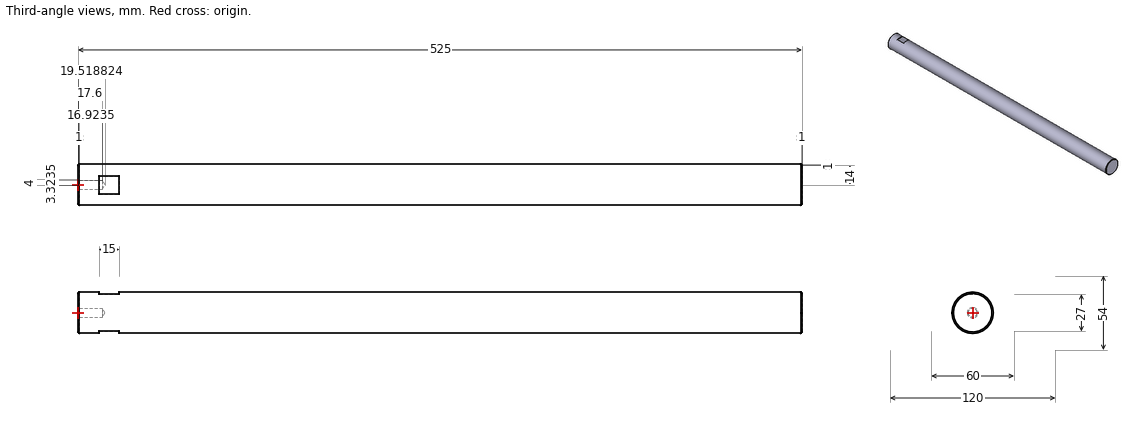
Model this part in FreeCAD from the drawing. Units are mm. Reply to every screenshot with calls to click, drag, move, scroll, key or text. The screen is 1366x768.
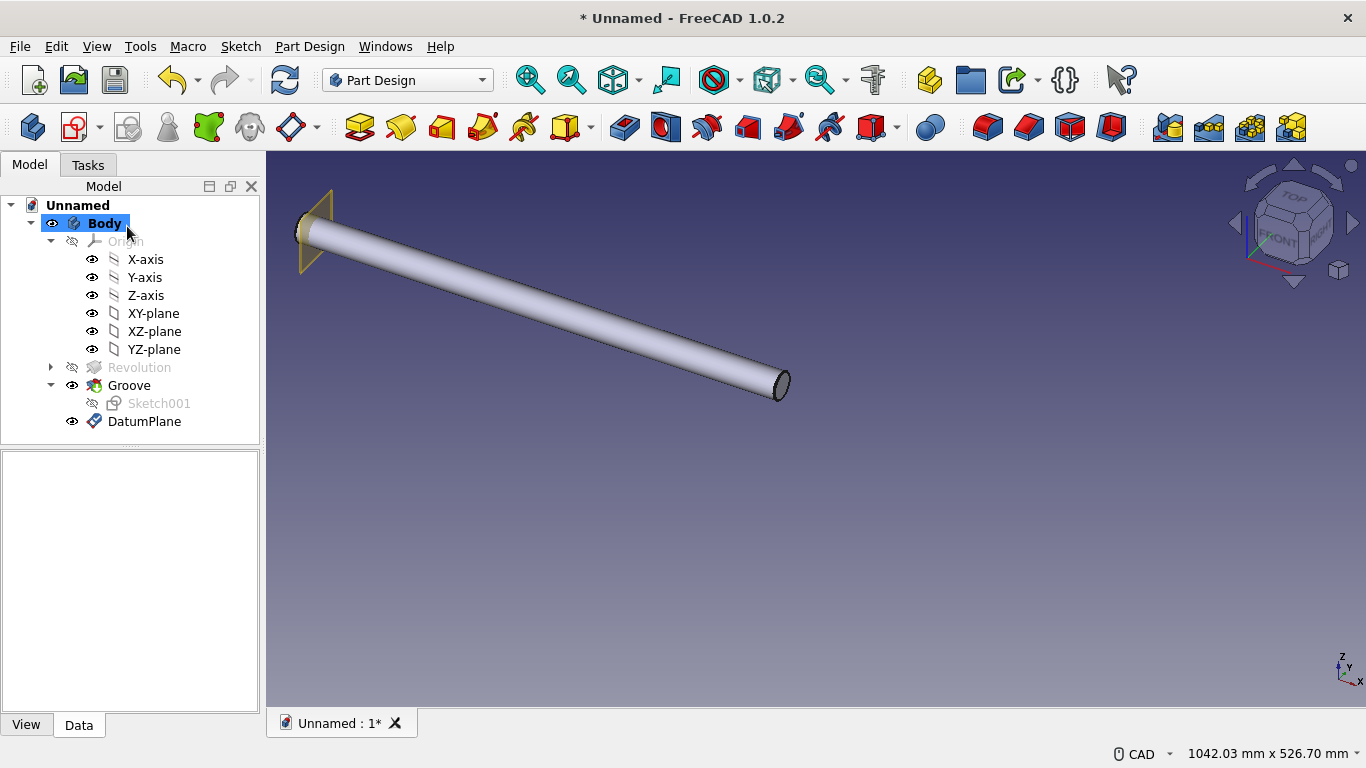
click(117, 421)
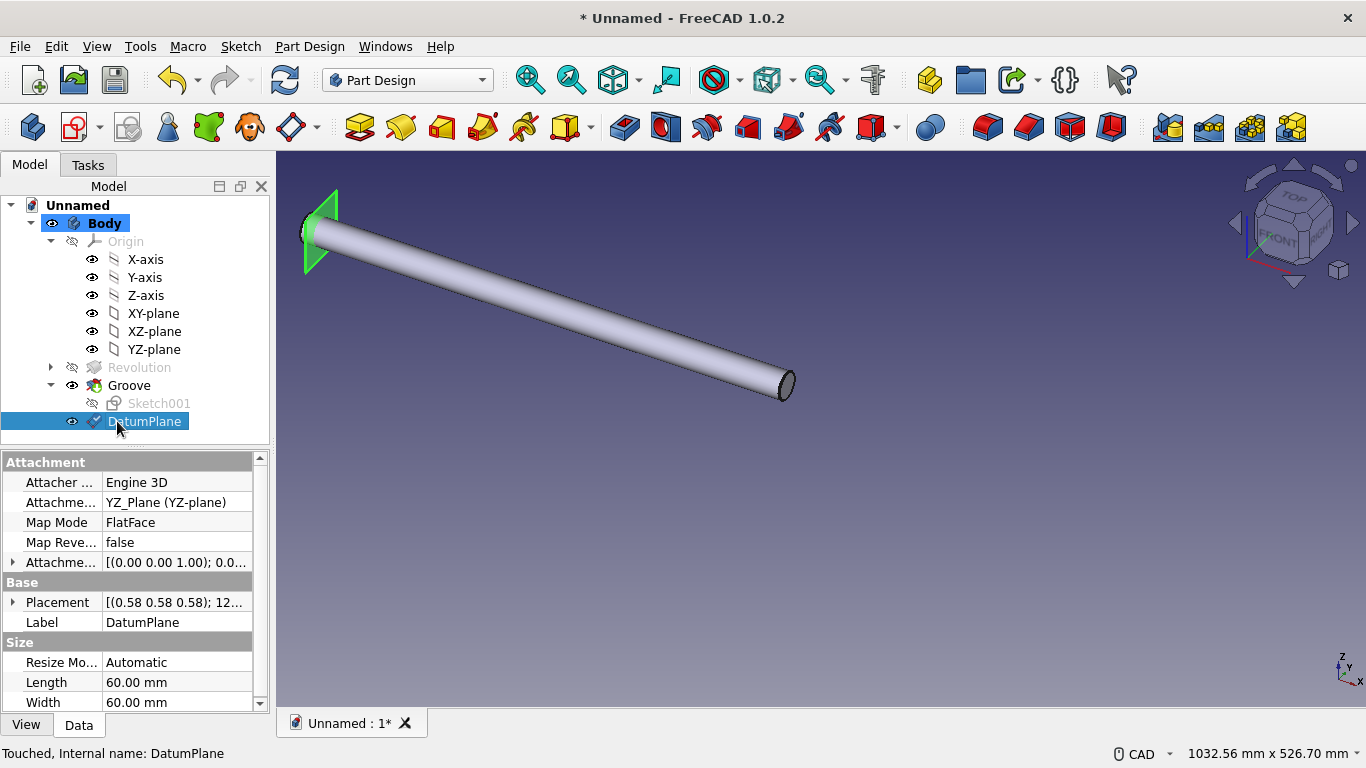
click(74, 128)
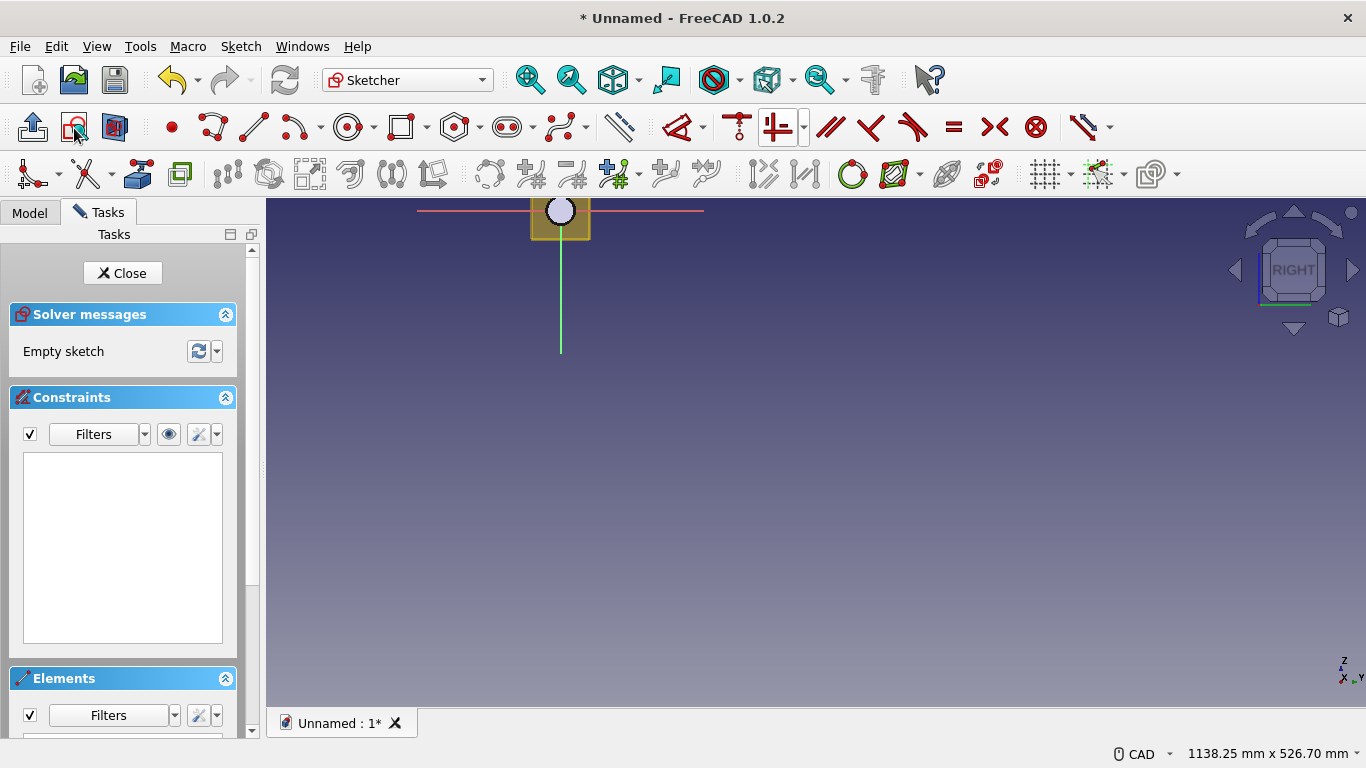
click(115, 128)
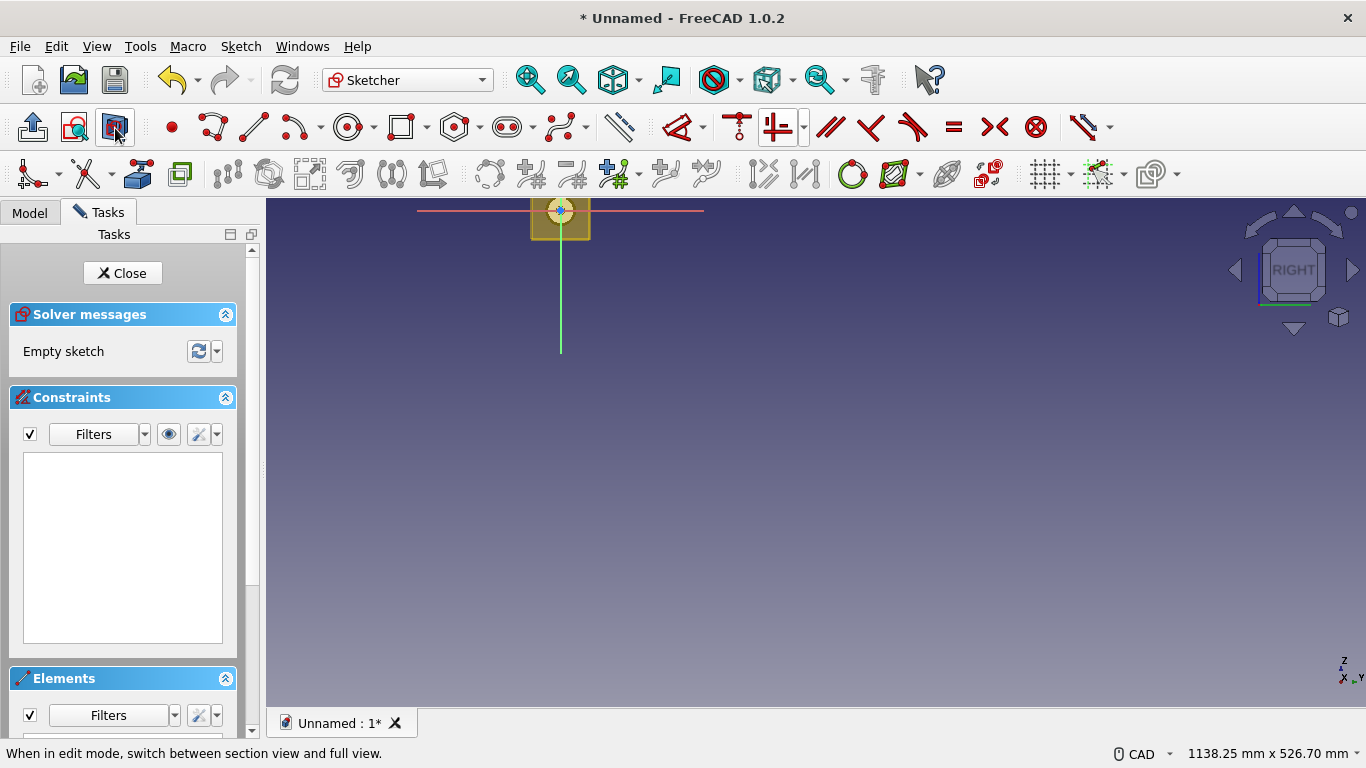
scroll(748, 452, down, 5)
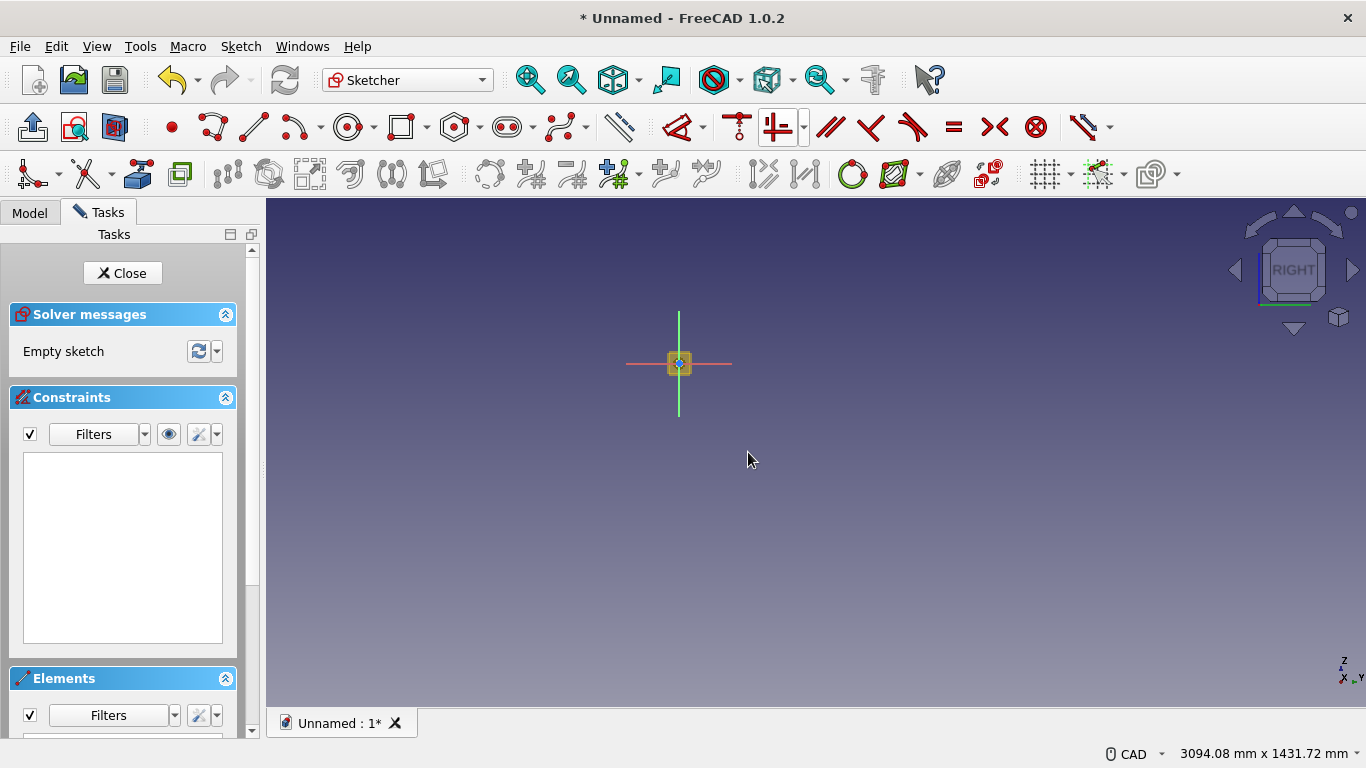
scroll(675, 358, up, 14)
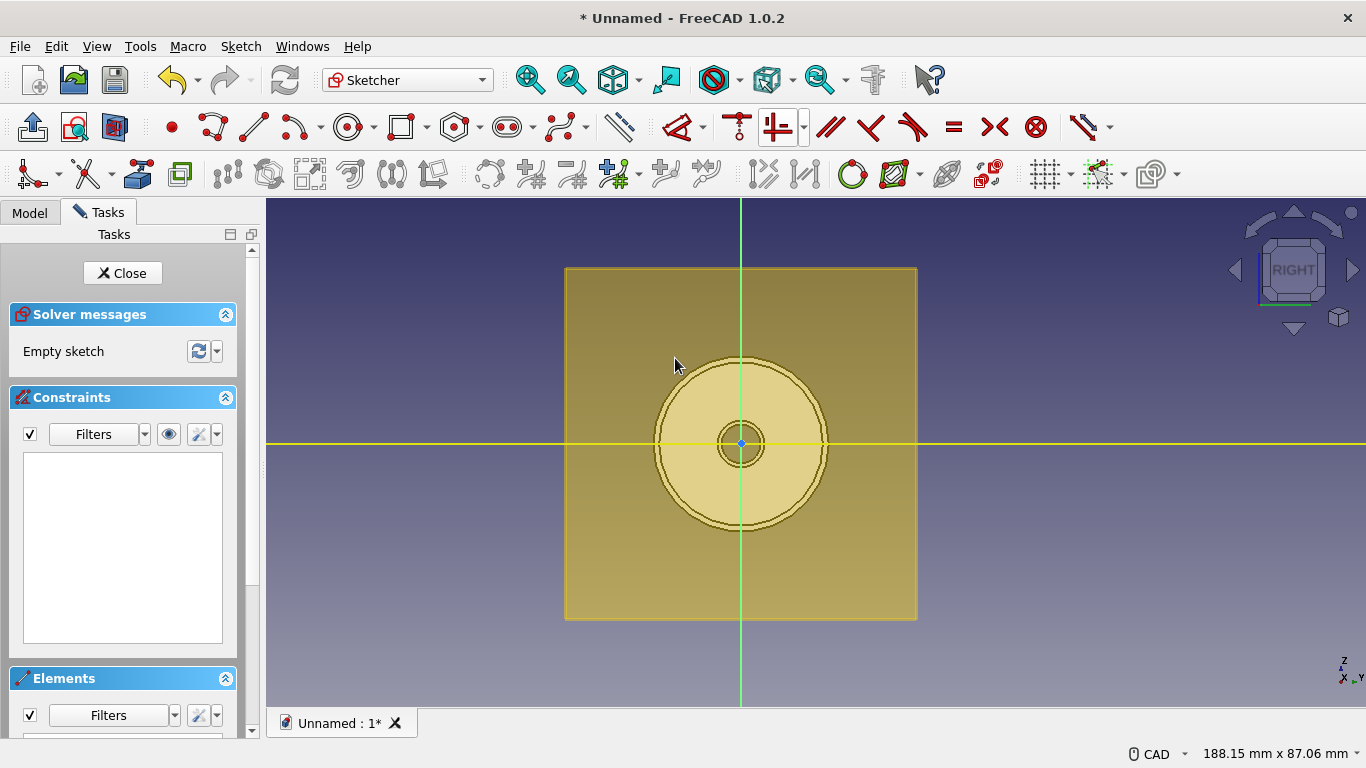
key(g)
key(v)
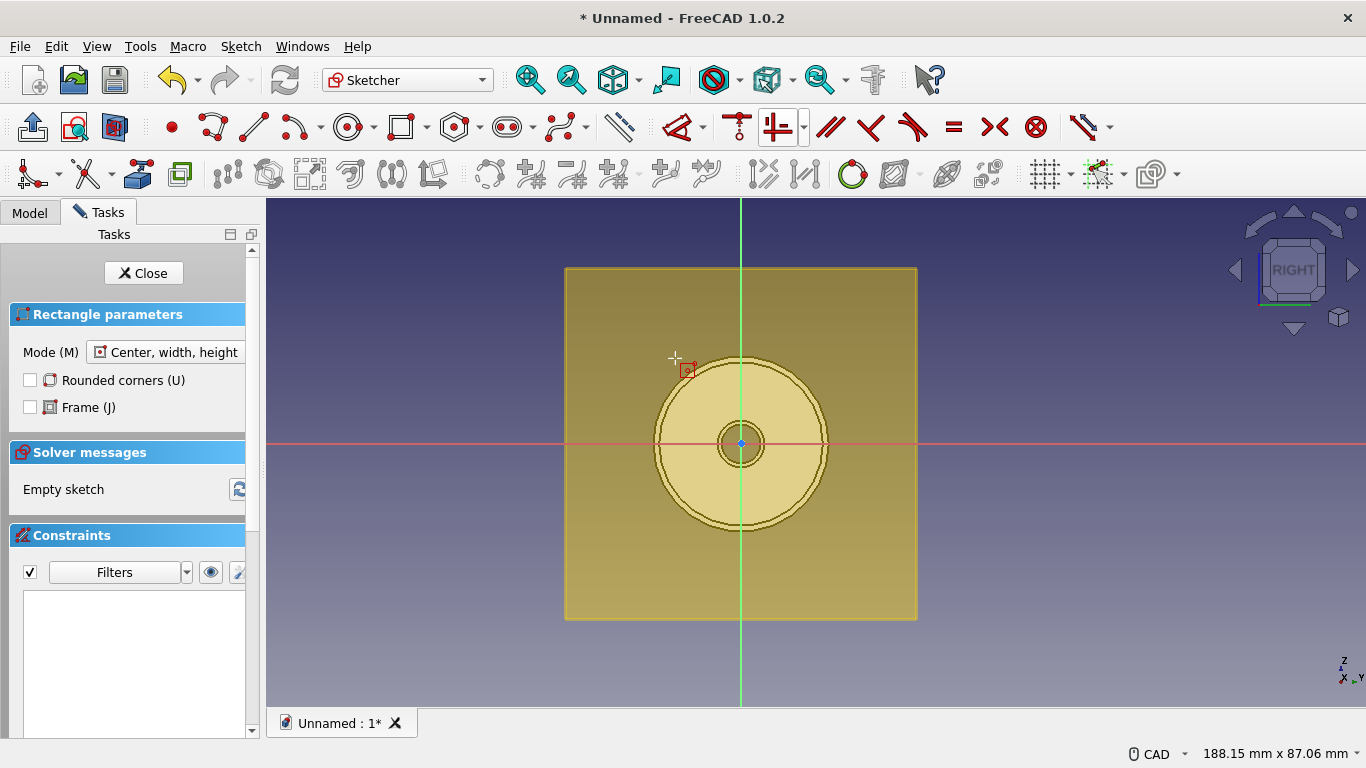
click(741, 444)
click(1092, 286)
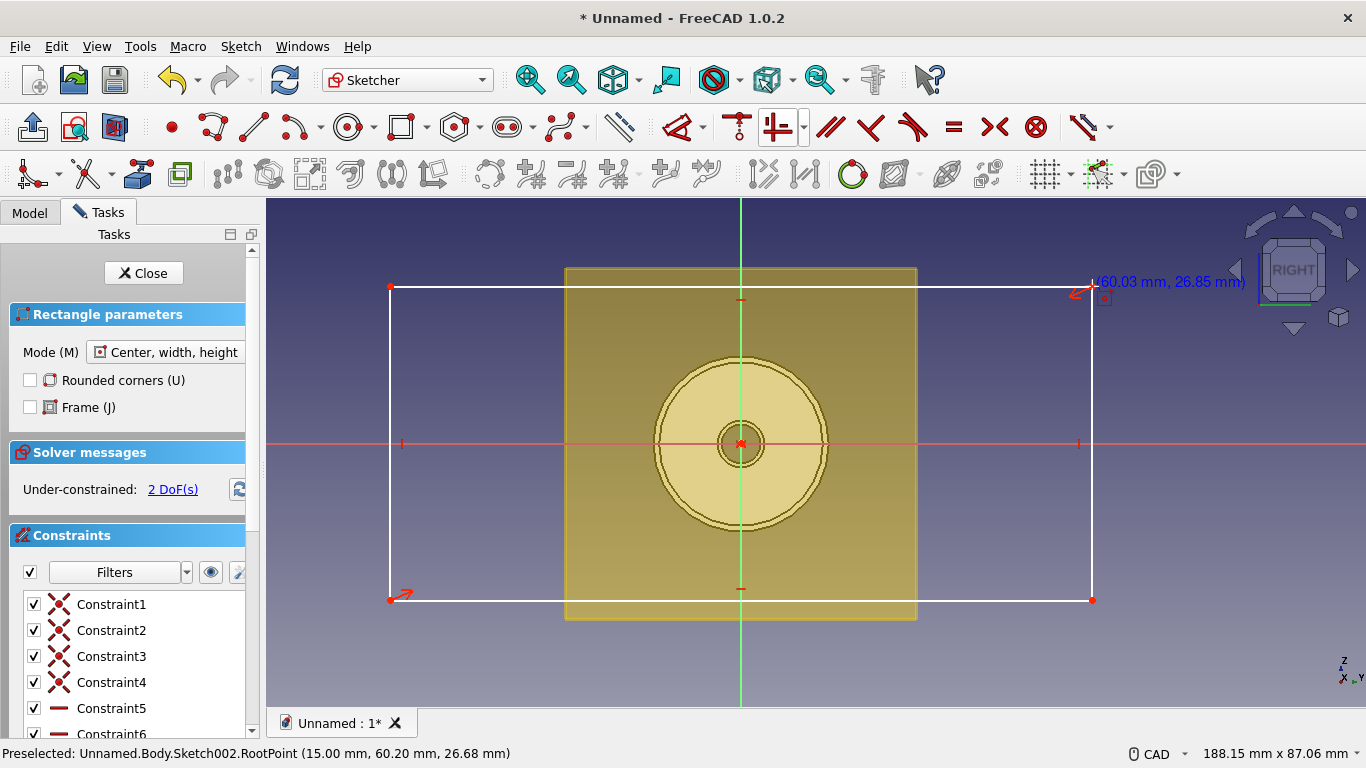
click(741, 444)
click(916, 365)
key(Escape)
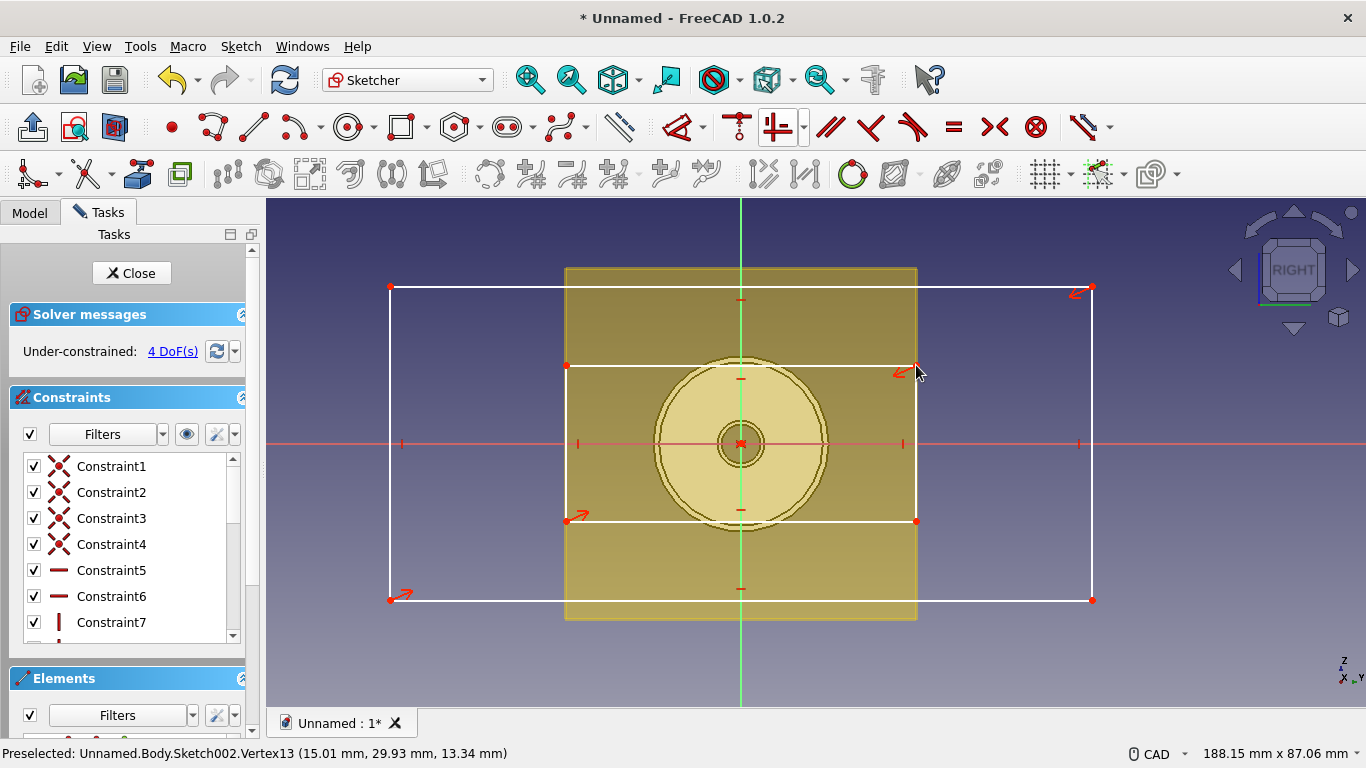
click(676, 128)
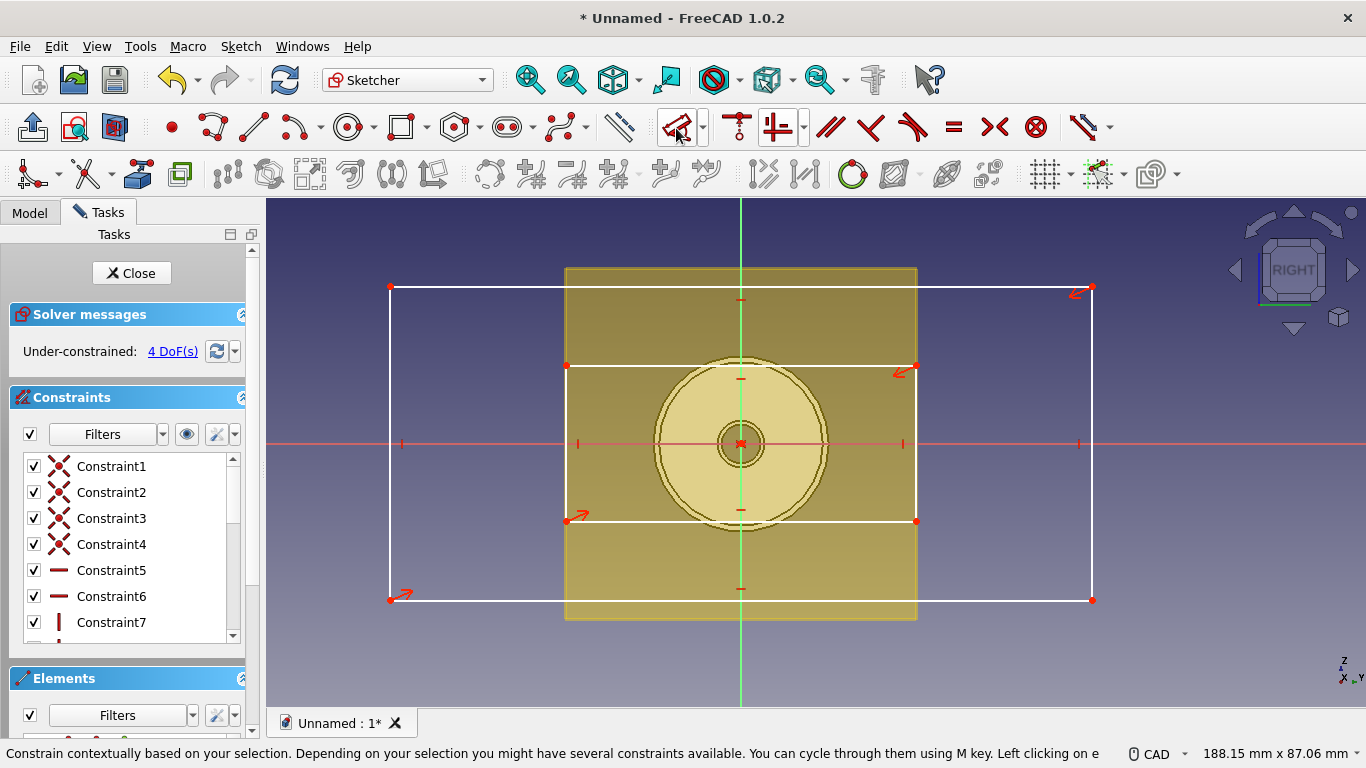
click(1092, 507)
click(1126, 372)